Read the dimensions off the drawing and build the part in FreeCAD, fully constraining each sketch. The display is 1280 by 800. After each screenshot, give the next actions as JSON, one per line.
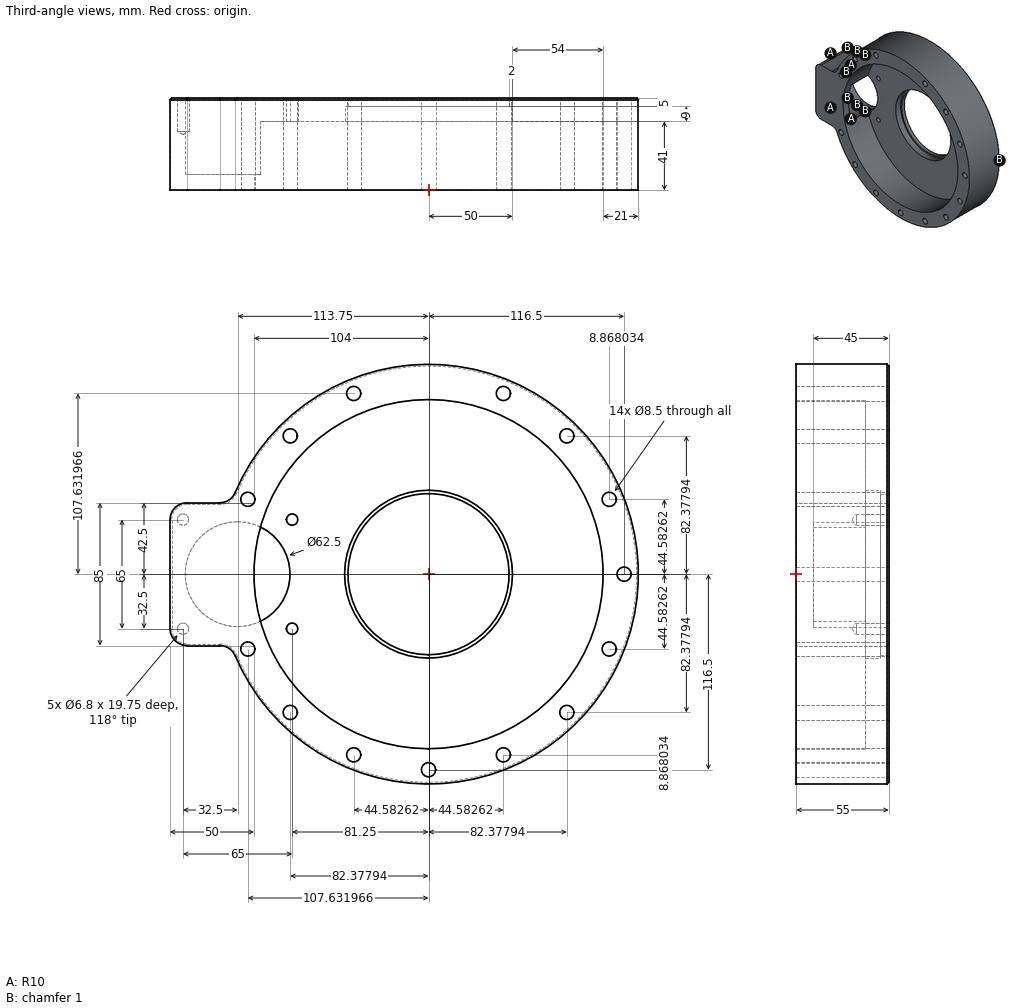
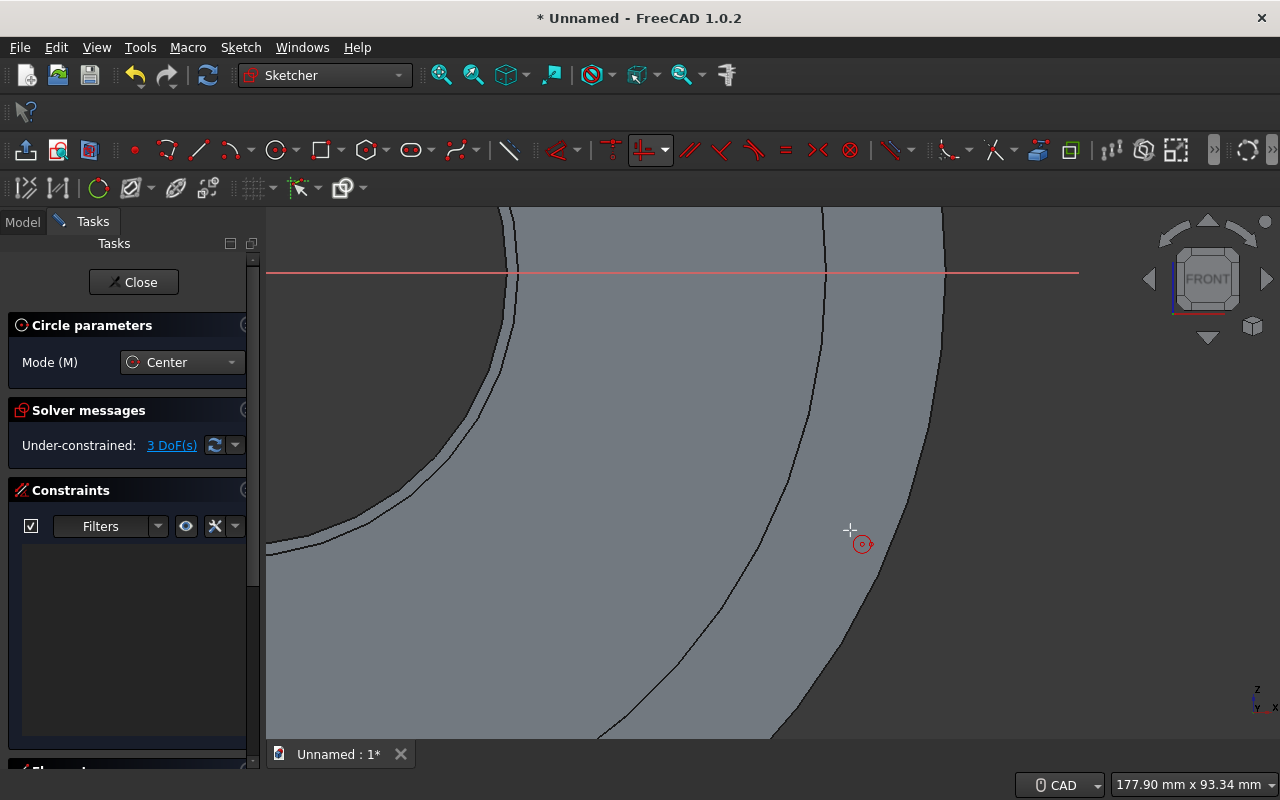
{"action": "scroll", "coordinate": [850, 530], "scroll_direction": "down", "scroll_amount": 7}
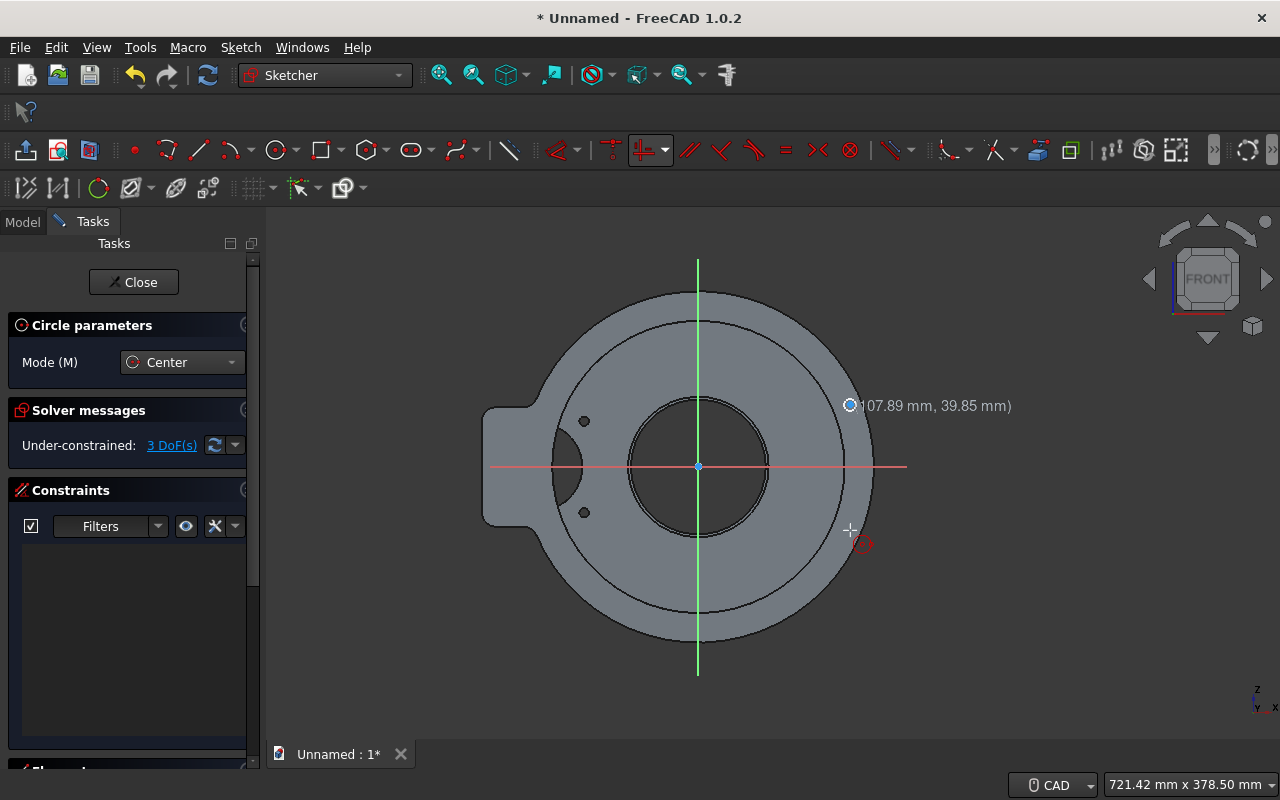
{"action": "left_click", "coordinate": [850, 530]}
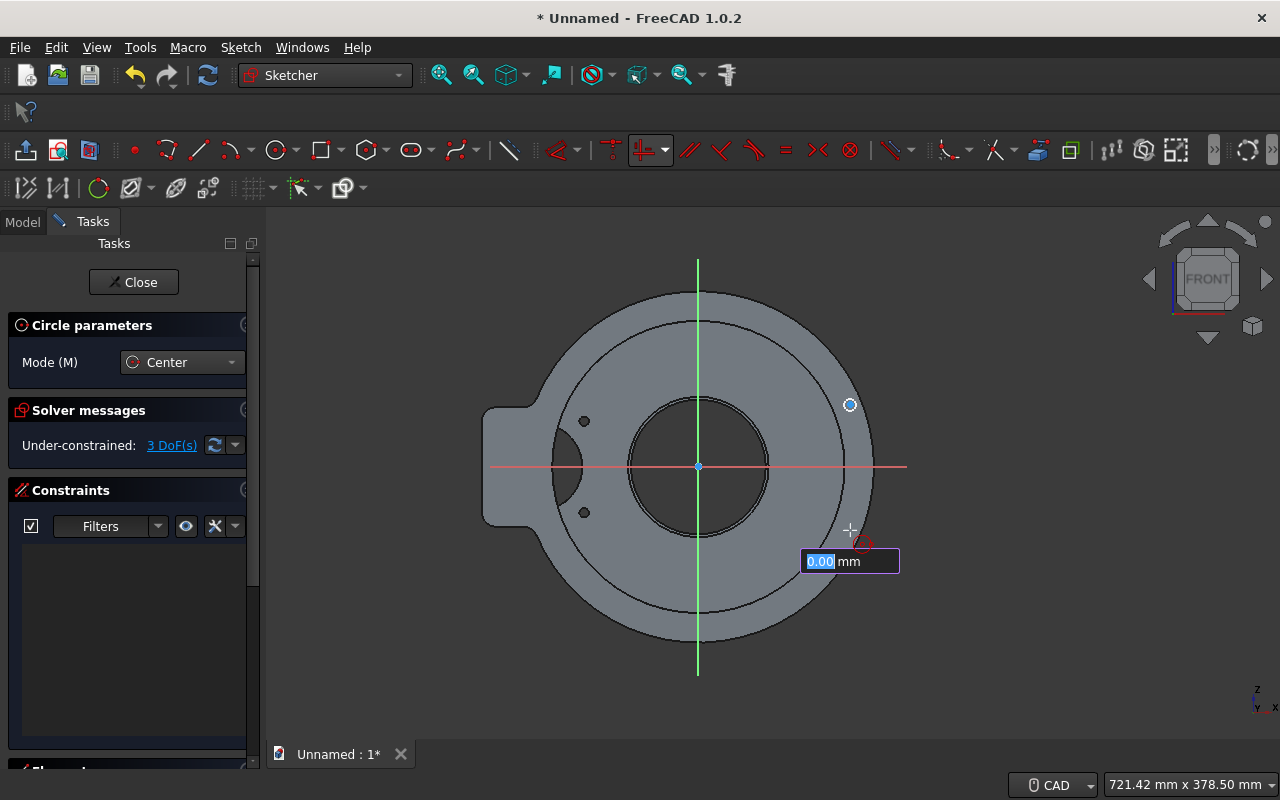
{"action": "scroll", "coordinate": [854, 525], "scroll_direction": "up", "scroll_amount": 5}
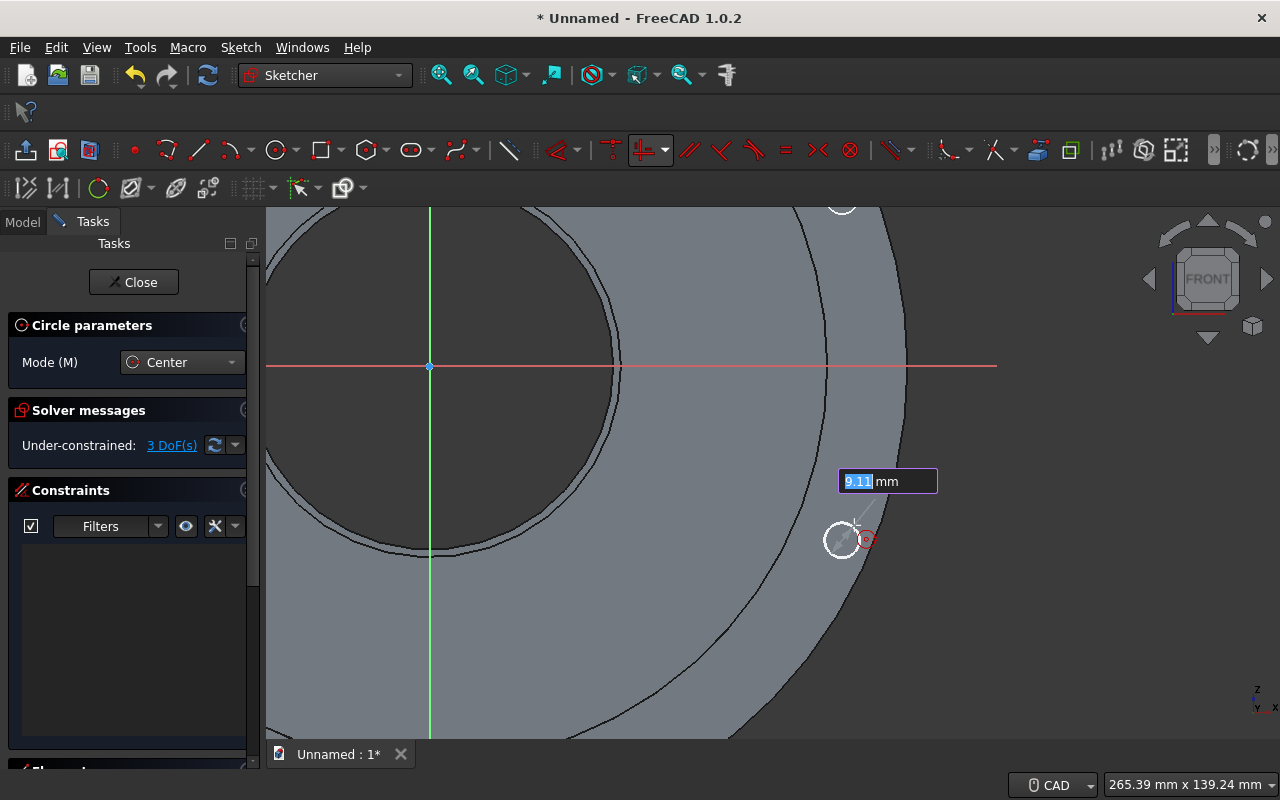
{"action": "left_click", "coordinate": [853, 525]}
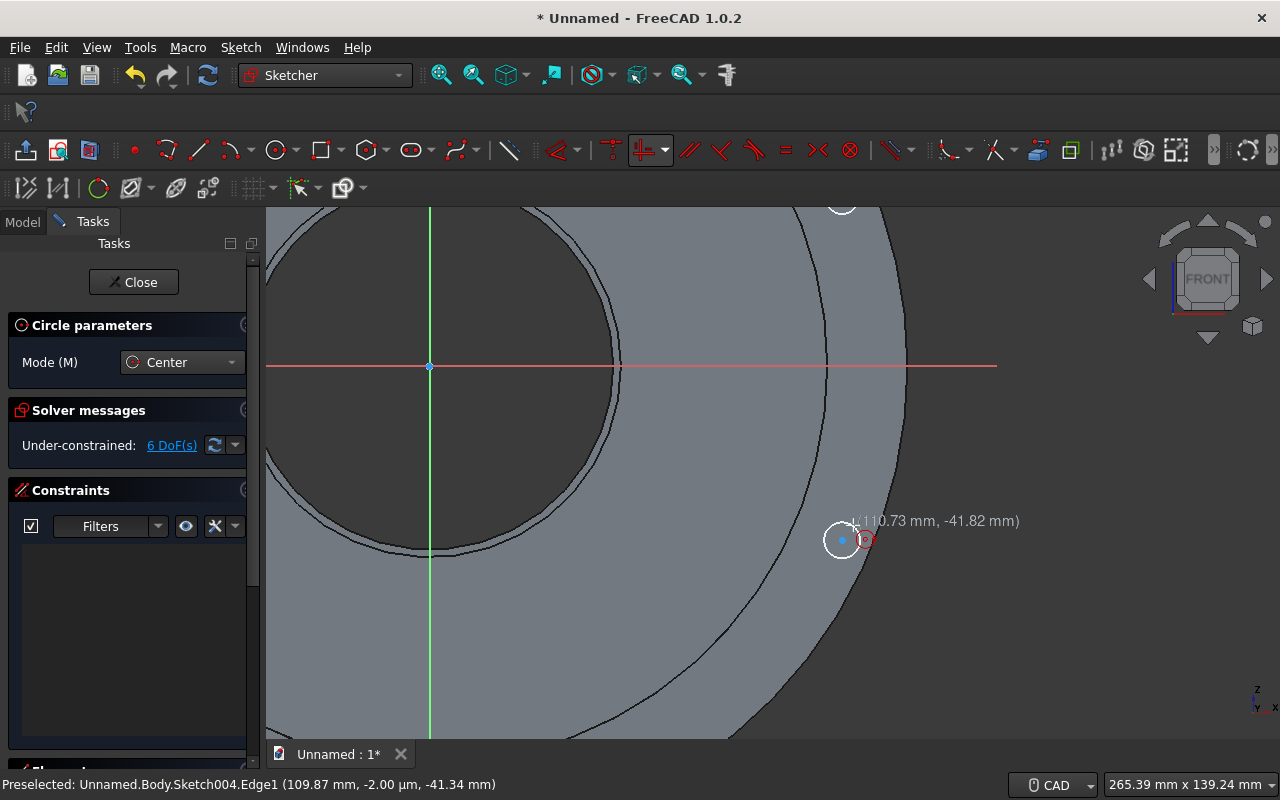
{"action": "scroll", "coordinate": [854, 525], "scroll_direction": "down", "scroll_amount": 5}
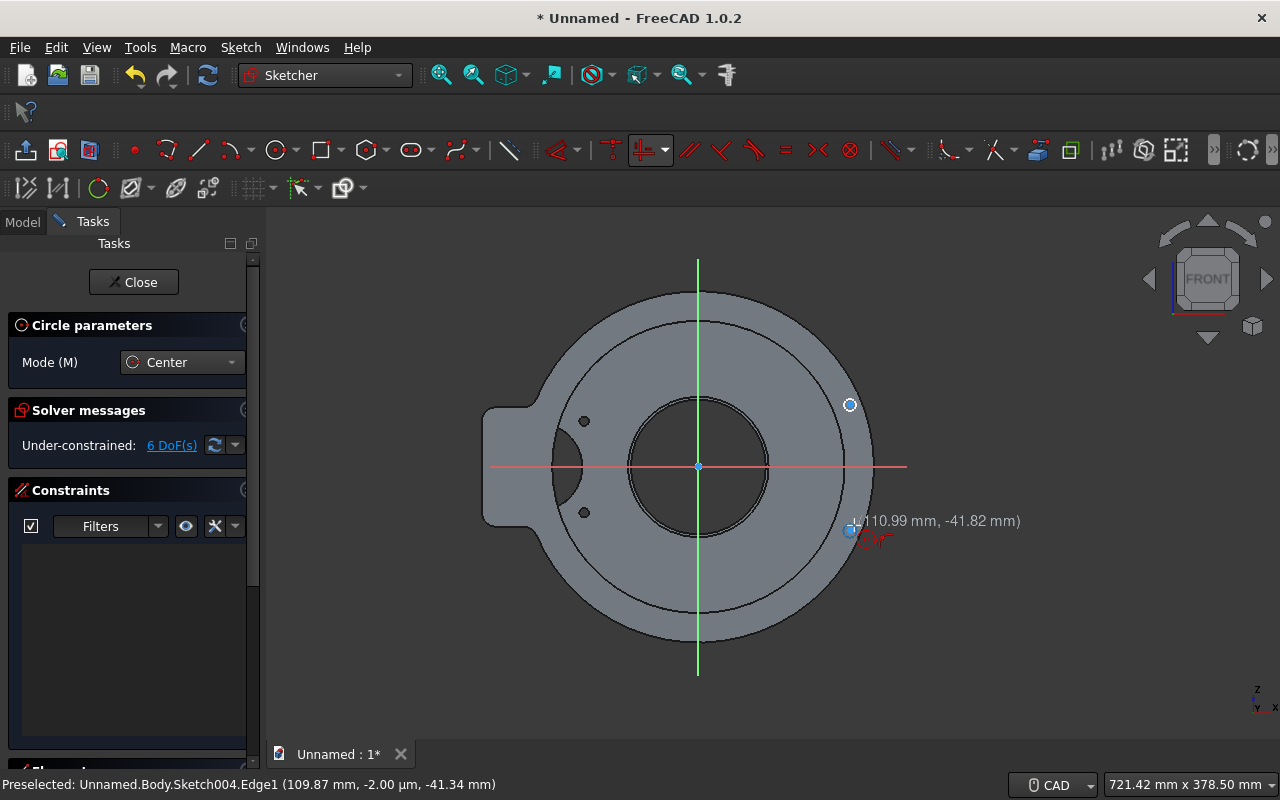
{"action": "scroll", "coordinate": [761, 618], "scroll_direction": "up", "scroll_amount": 7}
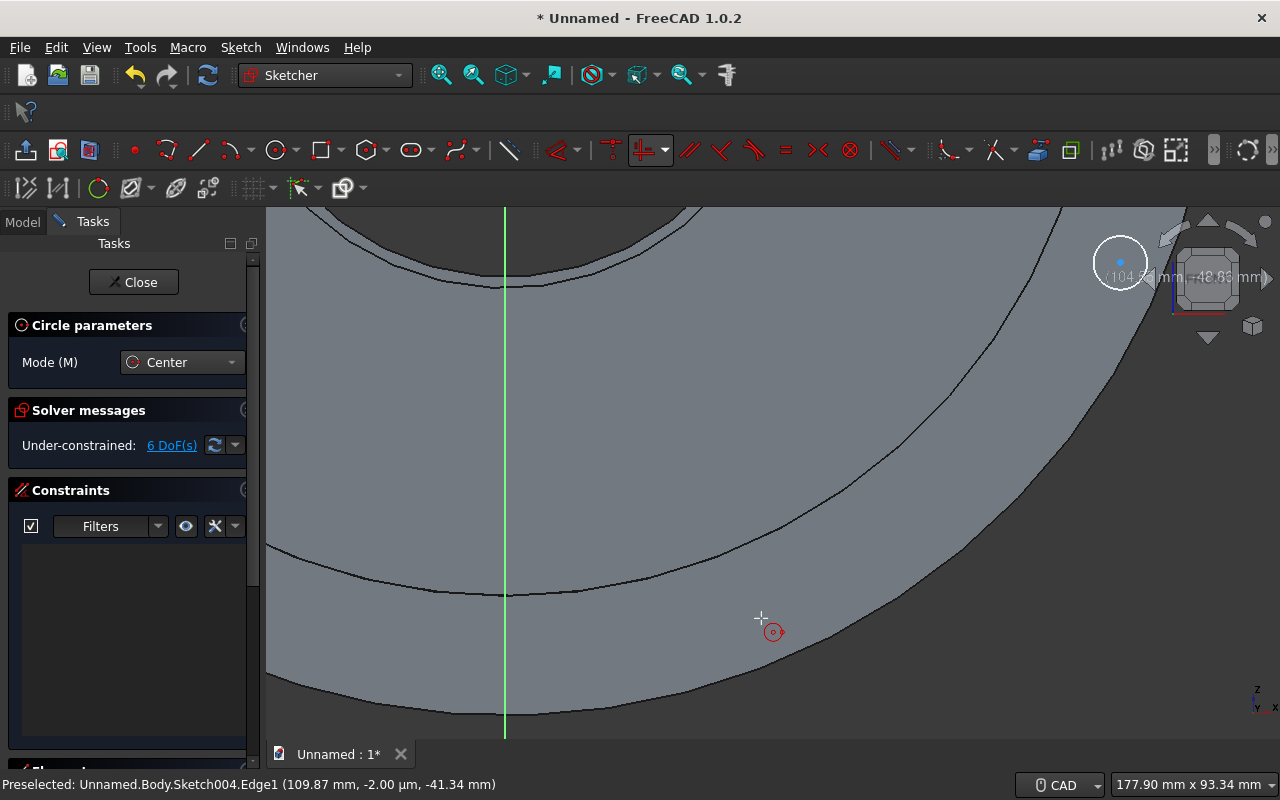
{"action": "scroll", "coordinate": [761, 619], "scroll_direction": "down", "scroll_amount": 7}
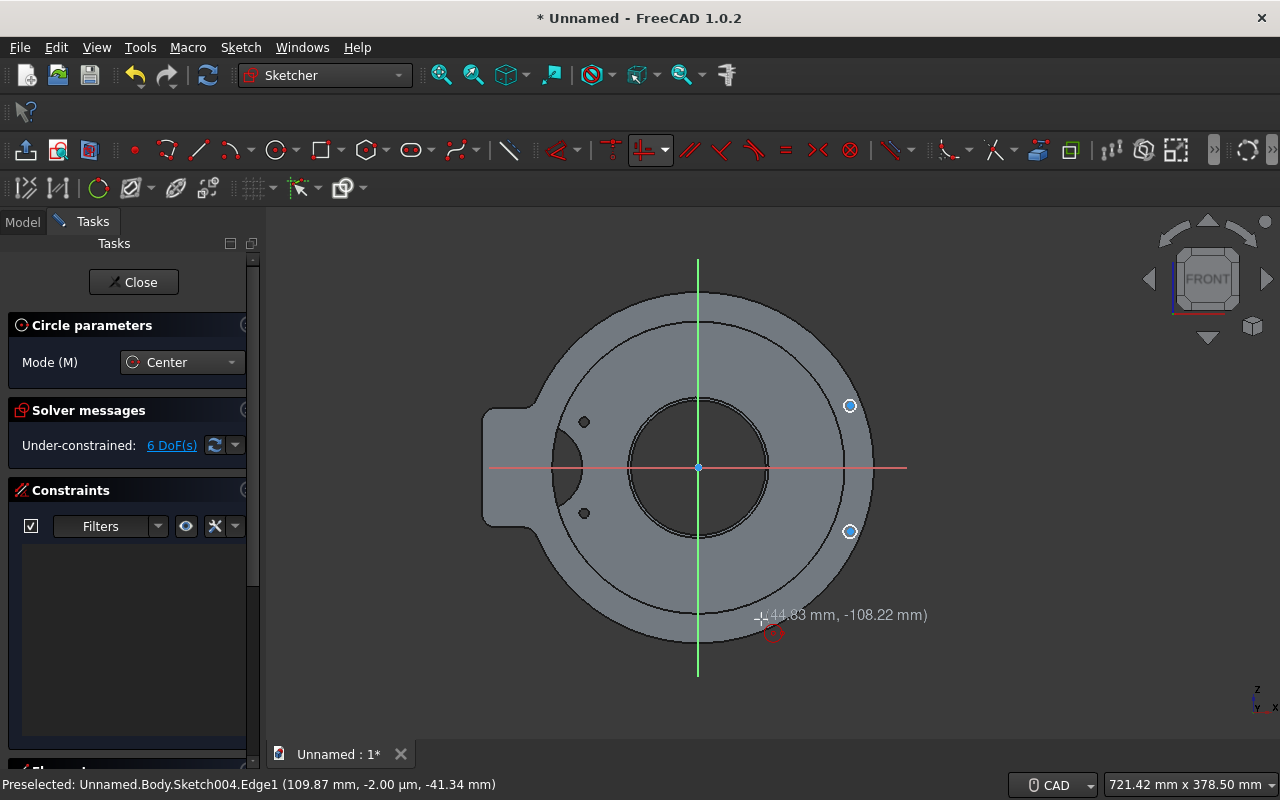
{"action": "left_click", "coordinate": [761, 619]}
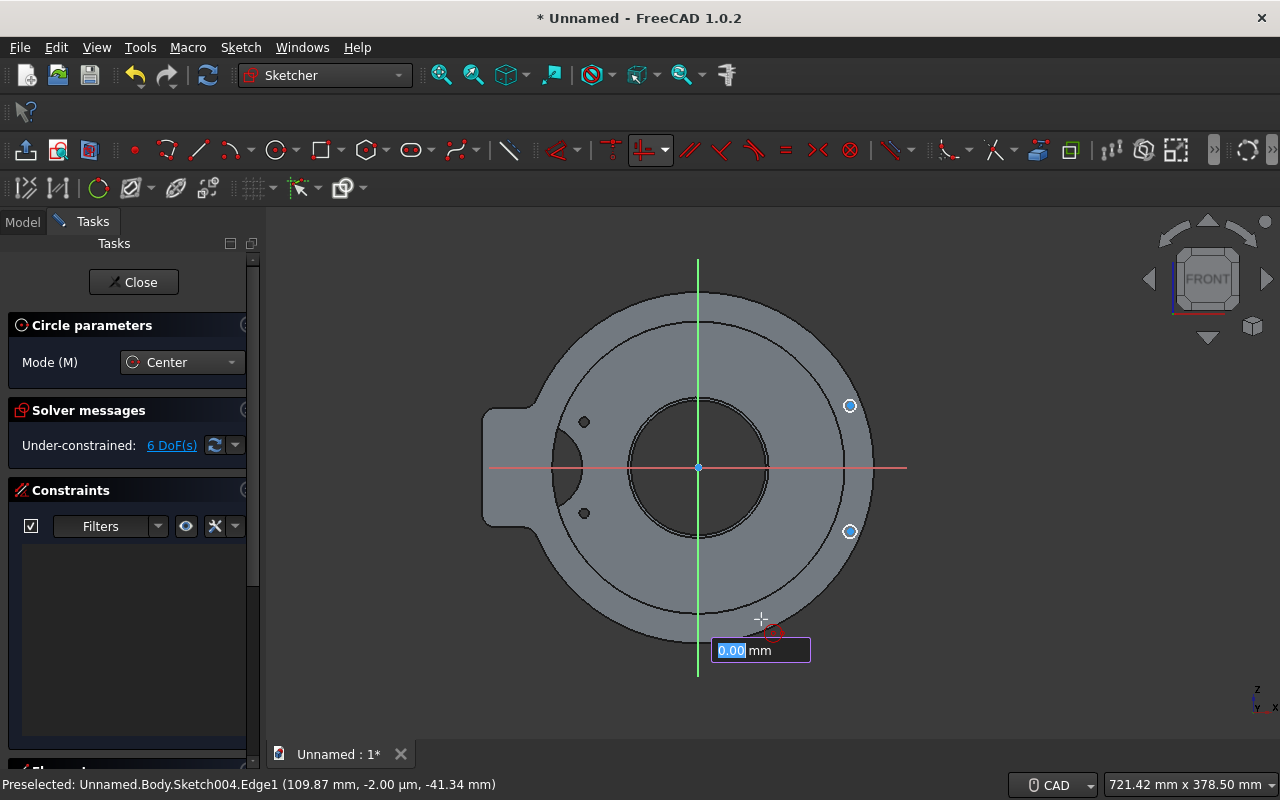
{"action": "scroll", "coordinate": [765, 615], "scroll_direction": "up", "scroll_amount": 5}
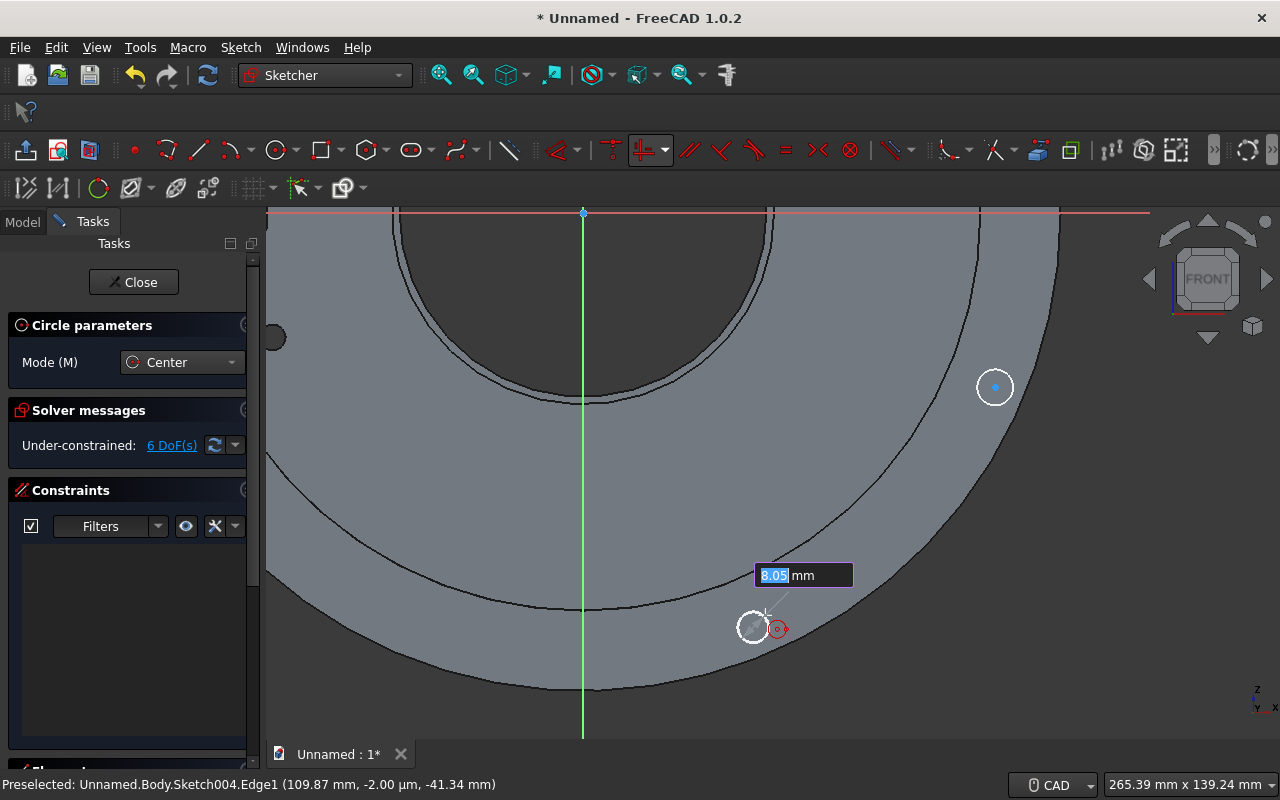
{"action": "left_click", "coordinate": [765, 613]}